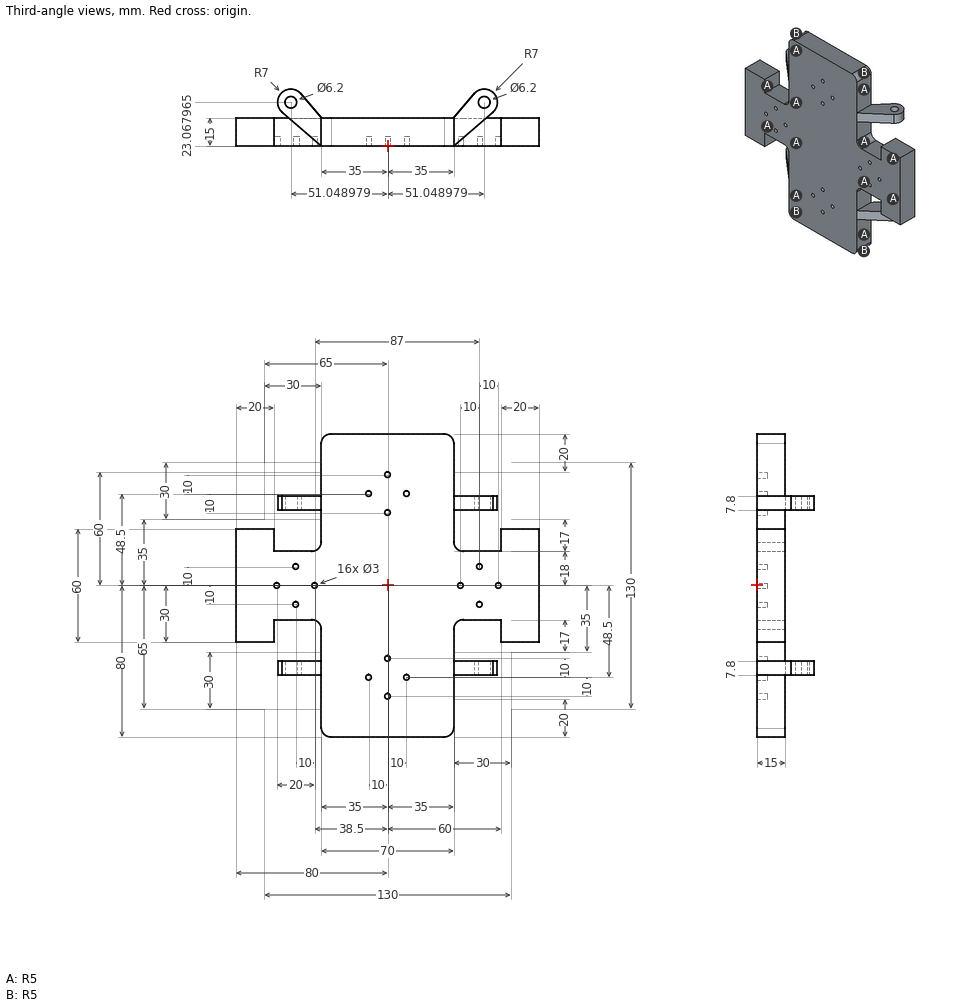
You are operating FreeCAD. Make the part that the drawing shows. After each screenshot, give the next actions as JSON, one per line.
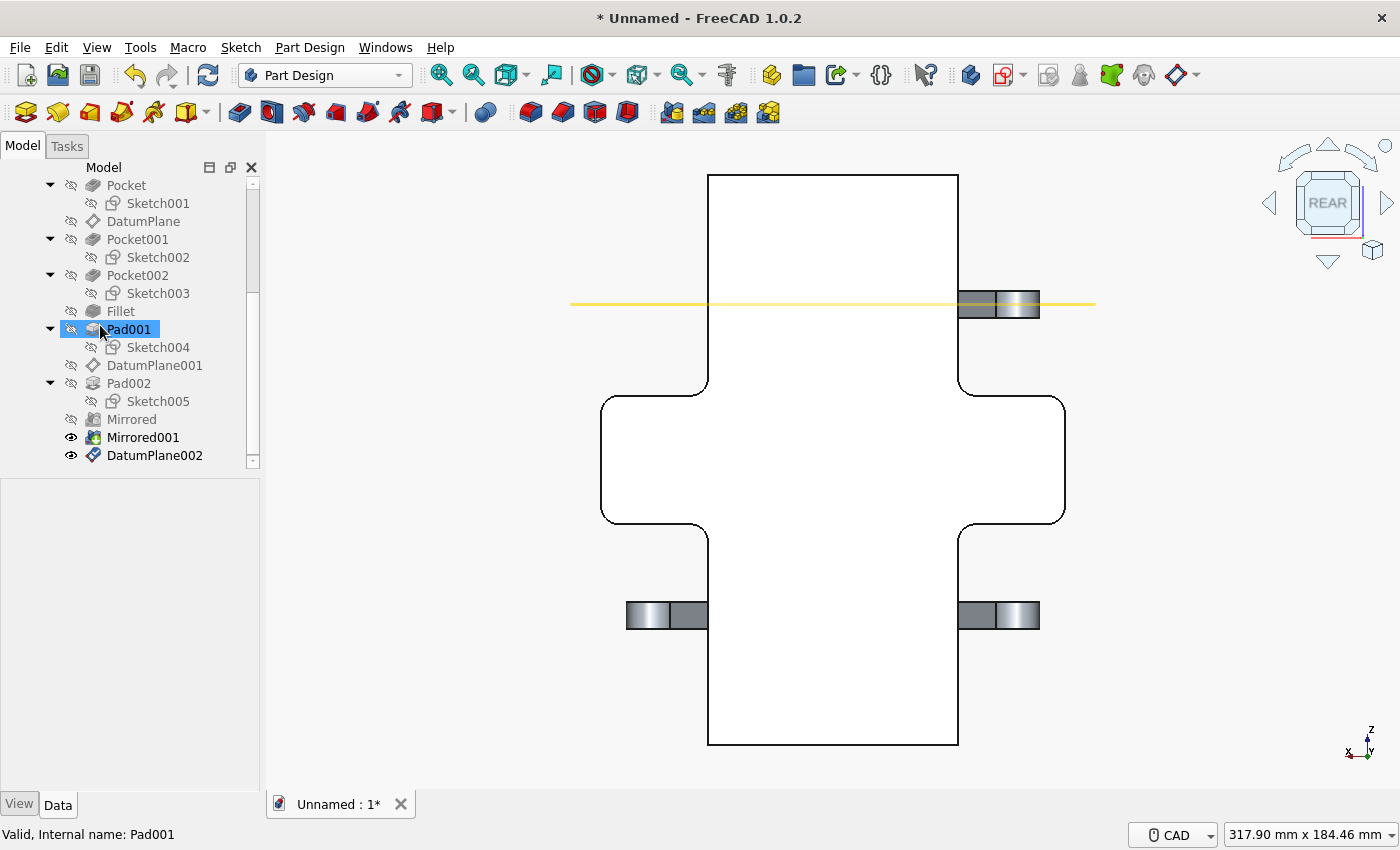
{"action": "left_click", "coordinate": [116, 455]}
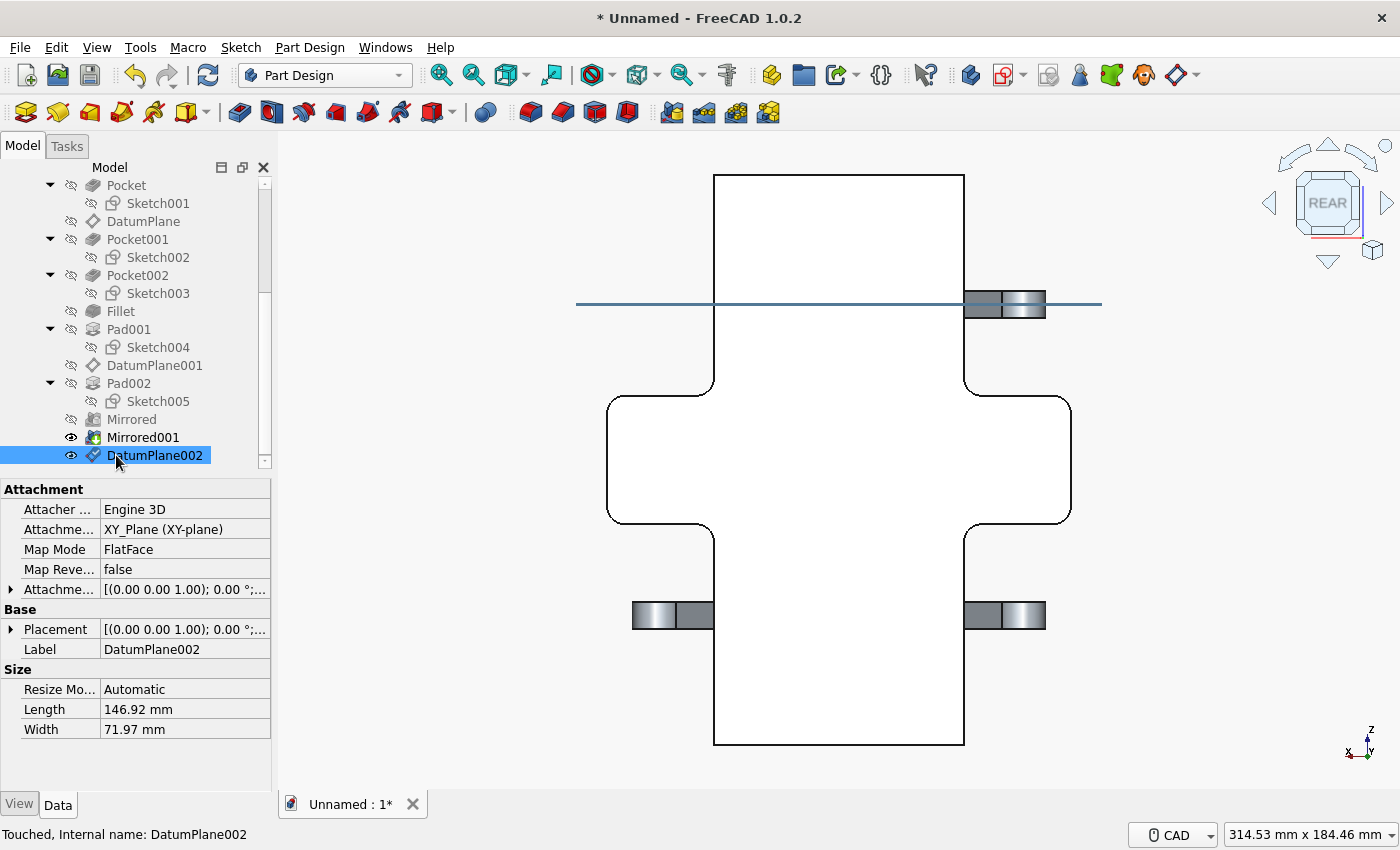
{"action": "left_click", "coordinate": [1004, 76]}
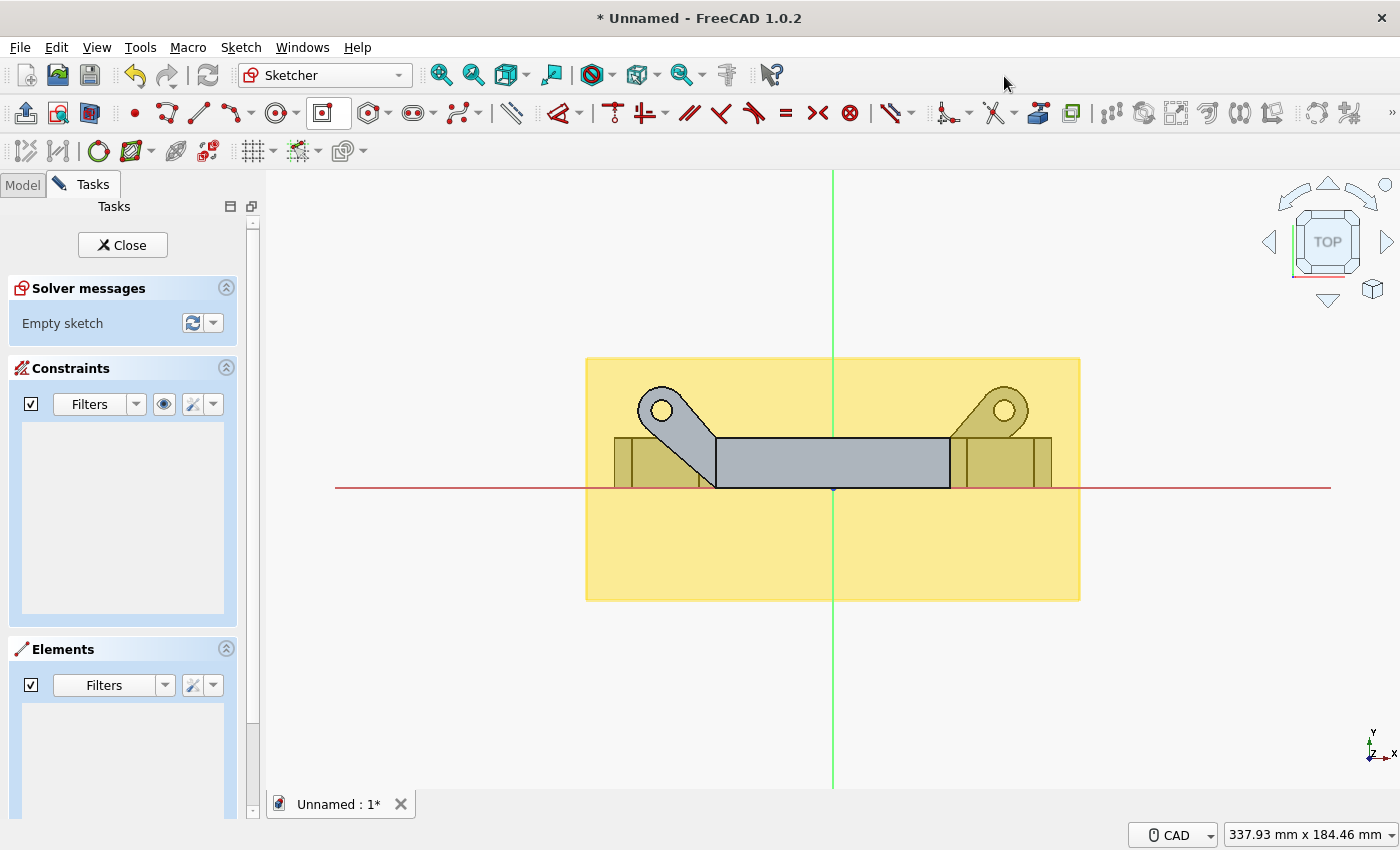
{"action": "key", "text": "q s"}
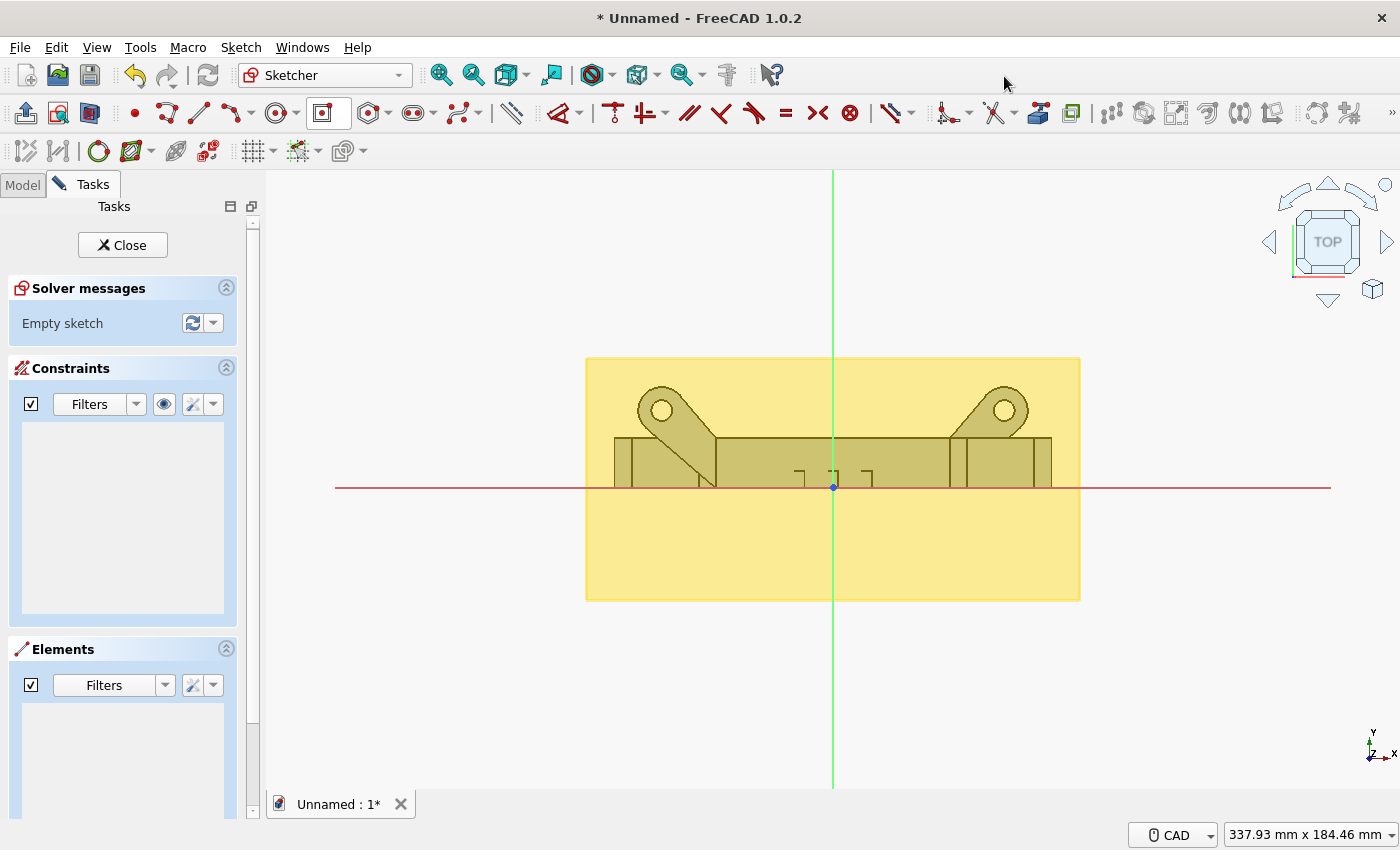
{"action": "scroll", "coordinate": [997, 424], "scroll_direction": "up", "scroll_amount": 6}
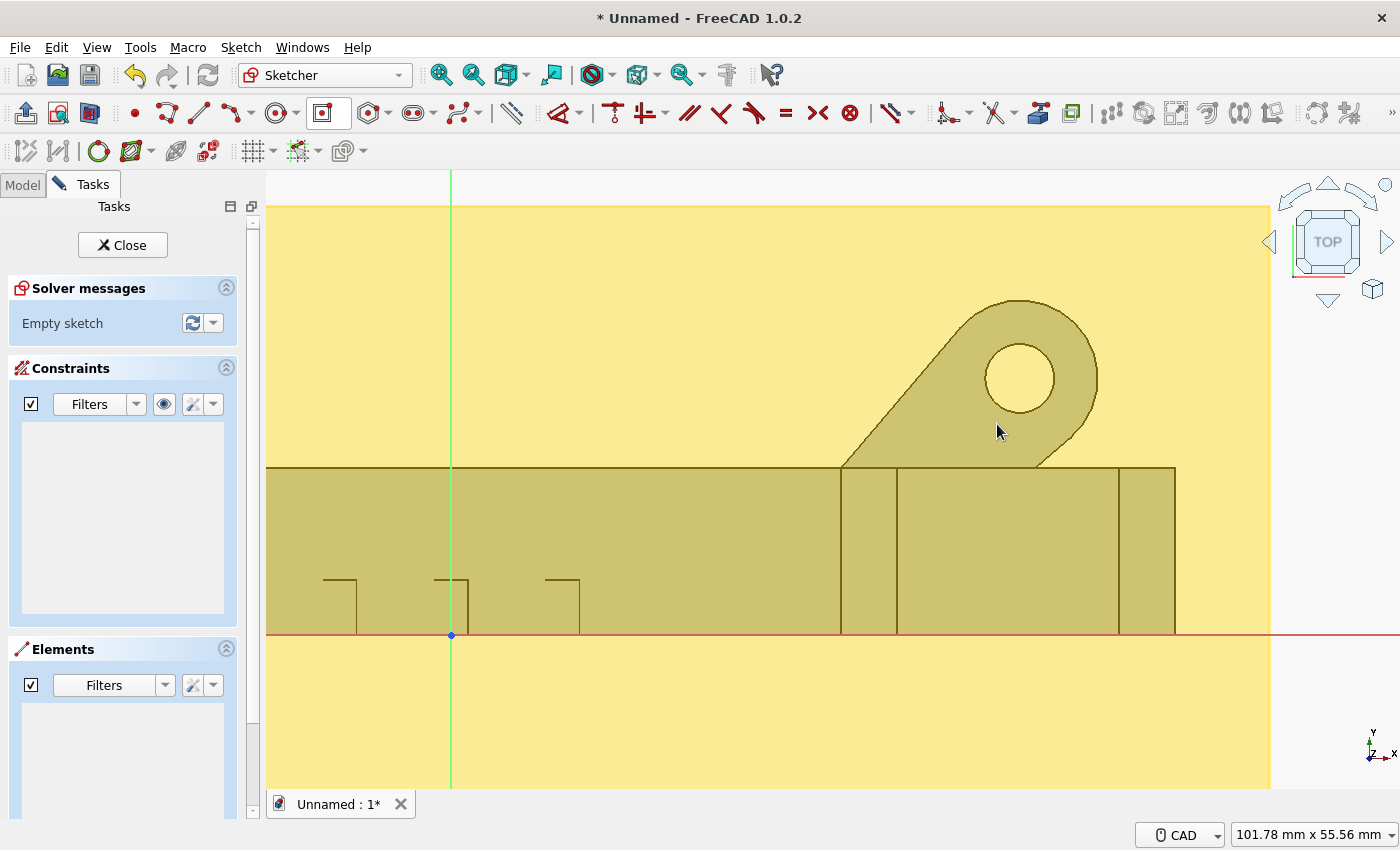
{"action": "key", "text": "g m"}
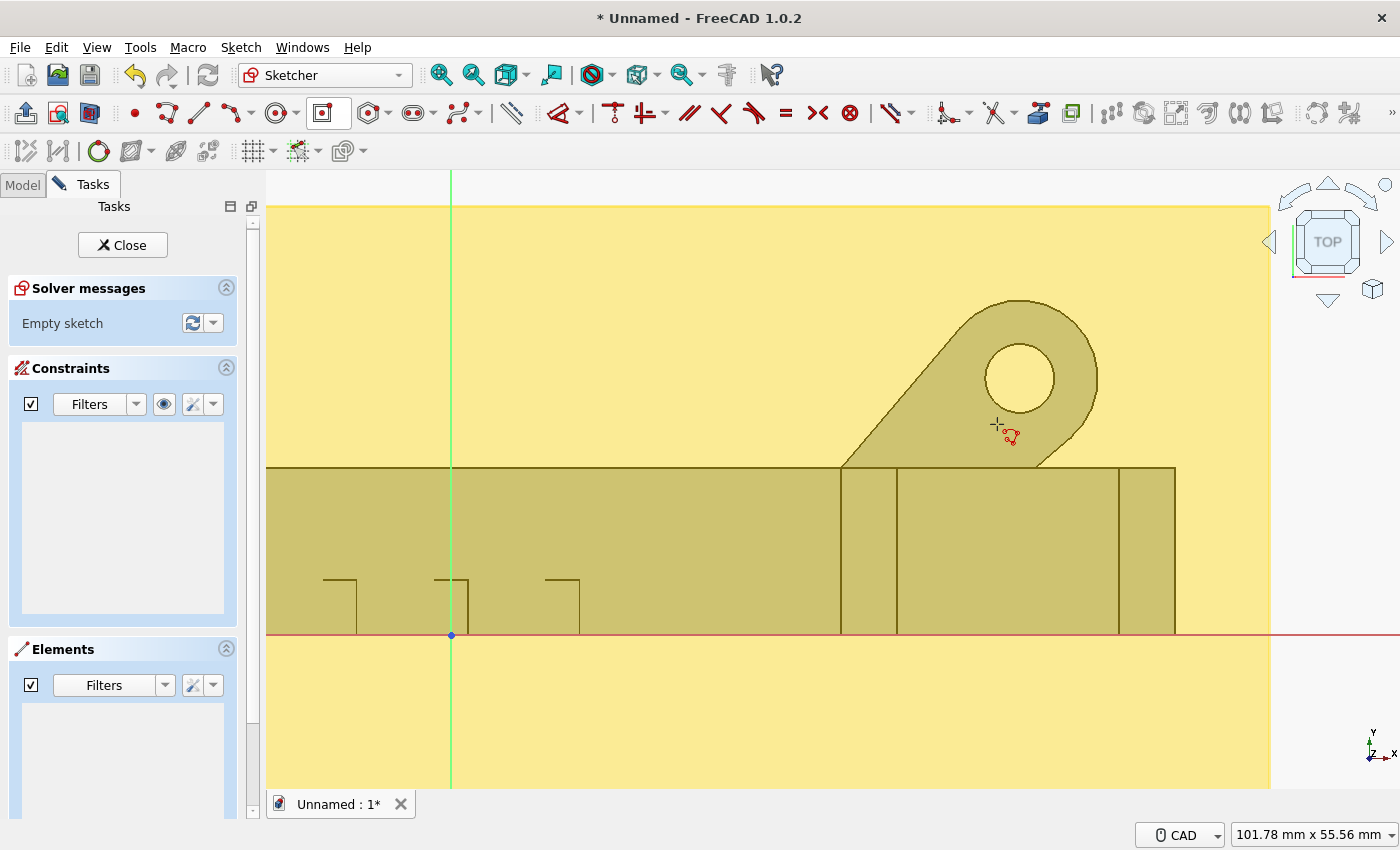
{"action": "left_click", "coordinate": [960, 328]}
{"action": "left_click", "coordinate": [841, 468]}
{"action": "left_click", "coordinate": [841, 635]}
{"action": "left_click", "coordinate": [1071, 438]}
{"action": "right_click", "coordinate": [1071, 438]}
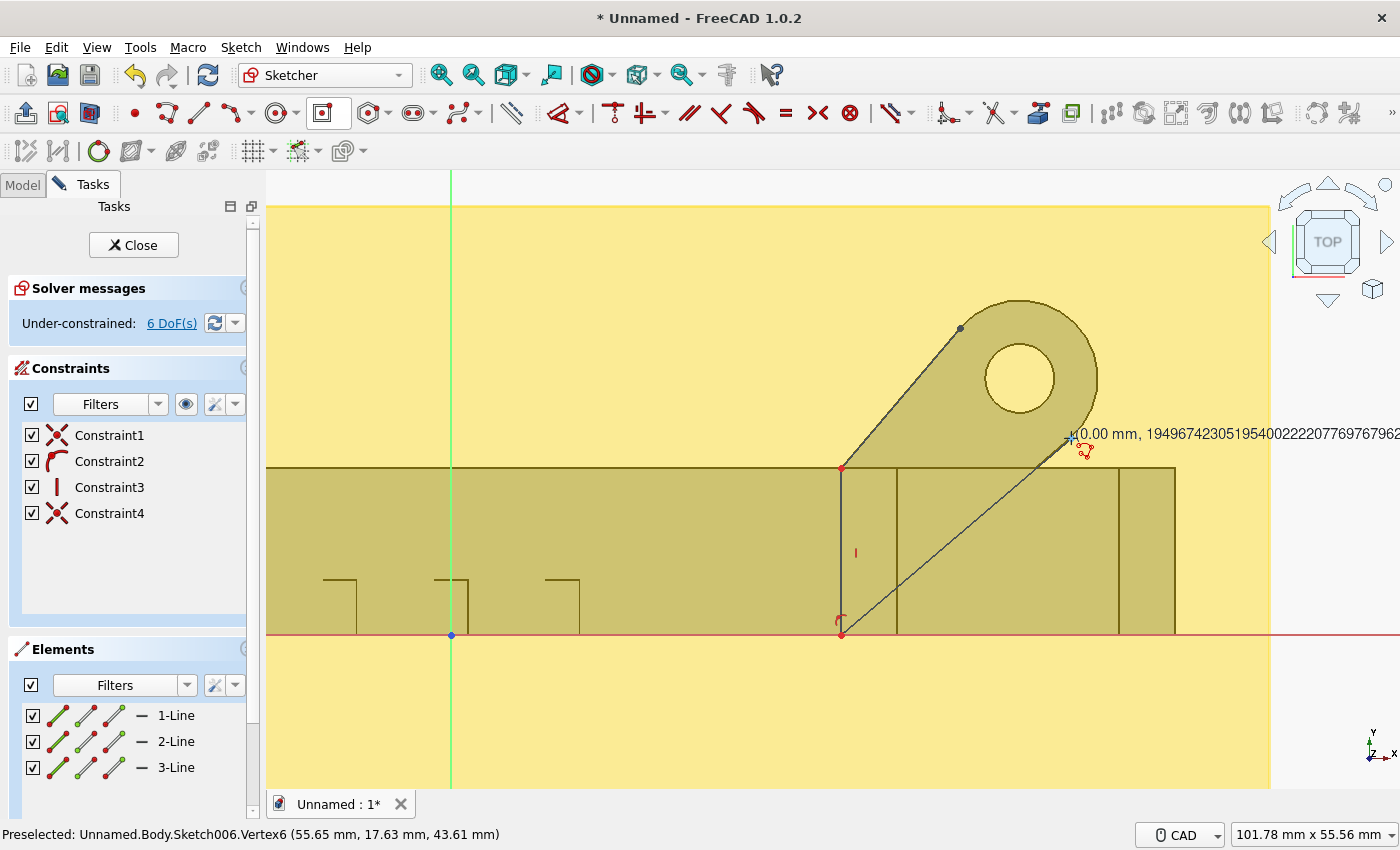
{"action": "key", "text": "g 3 a"}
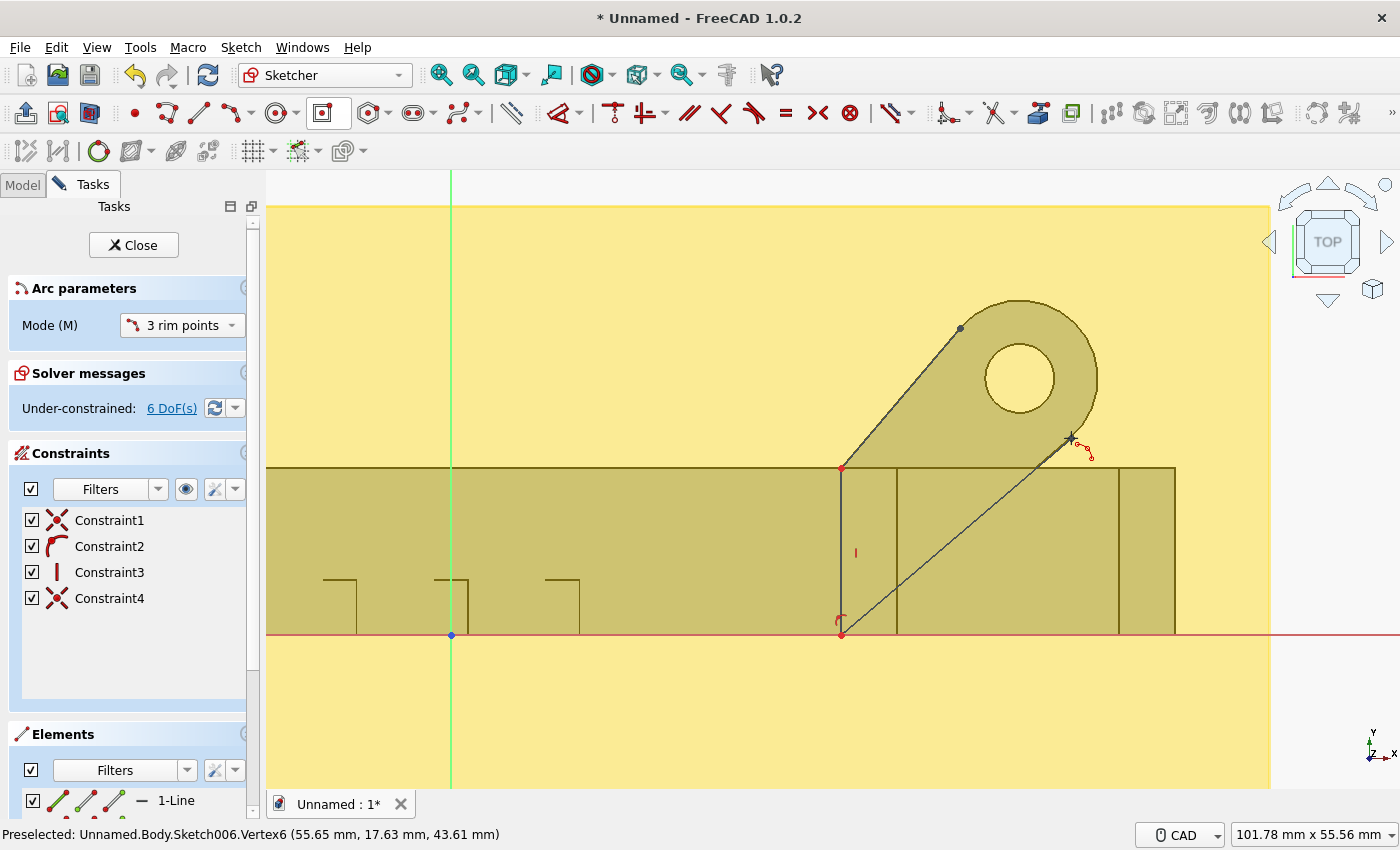
{"action": "left_click", "coordinate": [1071, 439]}
{"action": "left_click", "coordinate": [960, 329]}
{"action": "left_click", "coordinate": [1075, 323]}